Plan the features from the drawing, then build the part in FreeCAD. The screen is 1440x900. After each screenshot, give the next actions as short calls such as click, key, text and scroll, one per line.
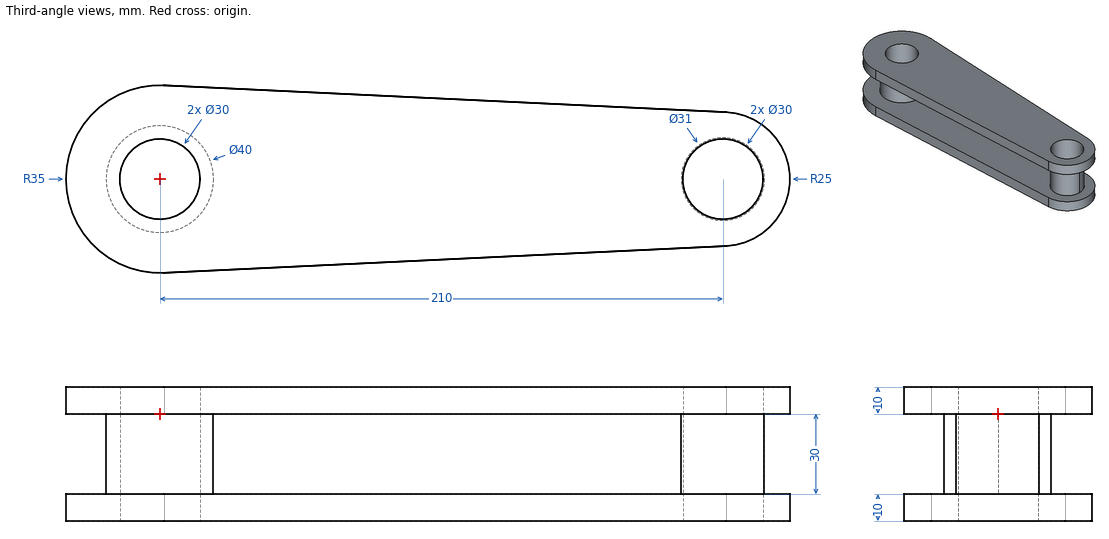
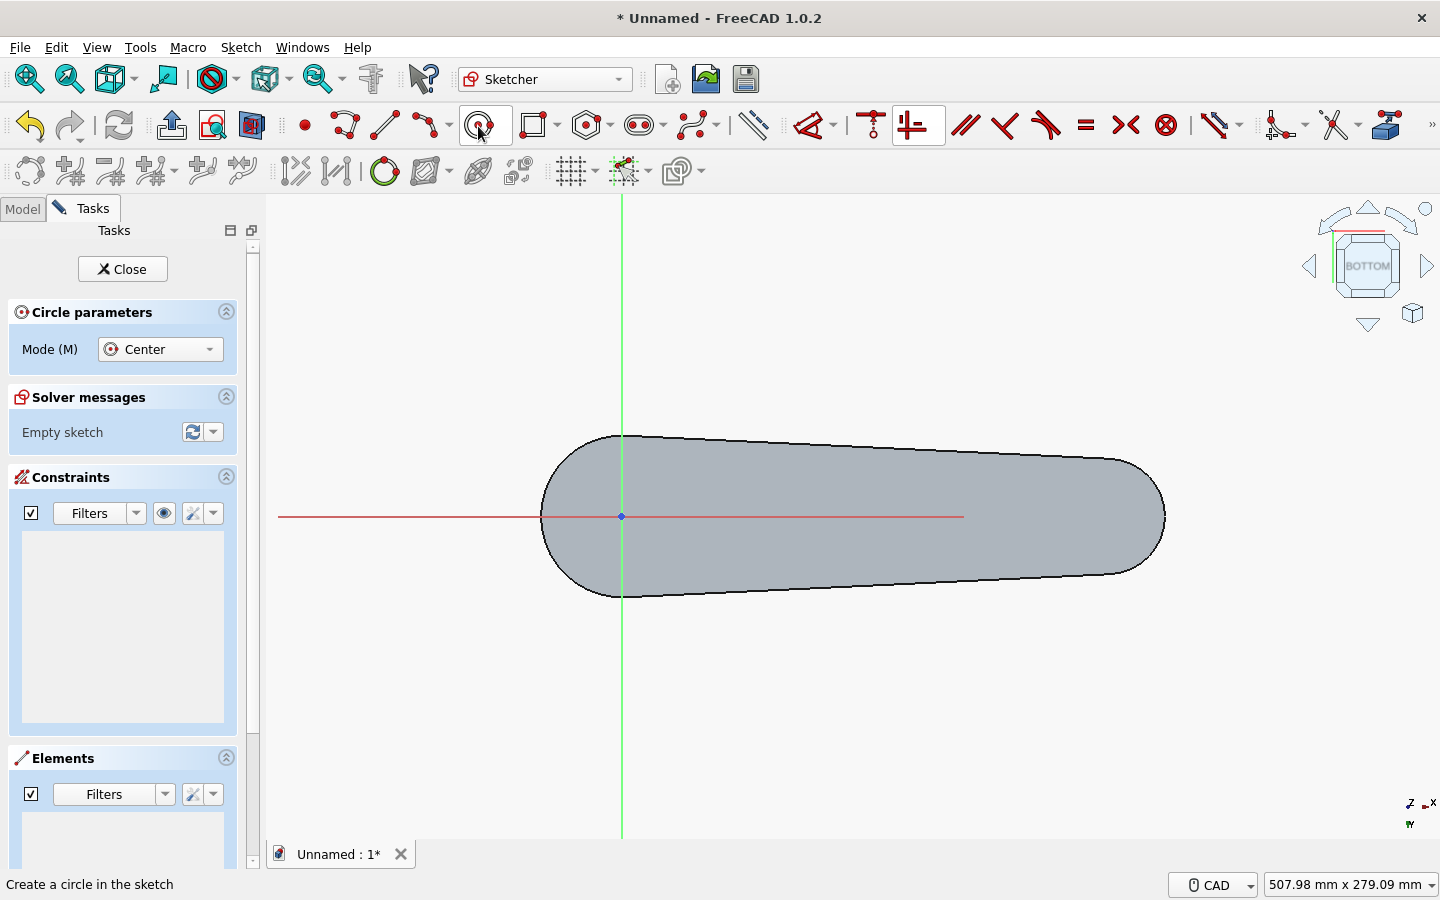
click(622, 516)
move(655, 484)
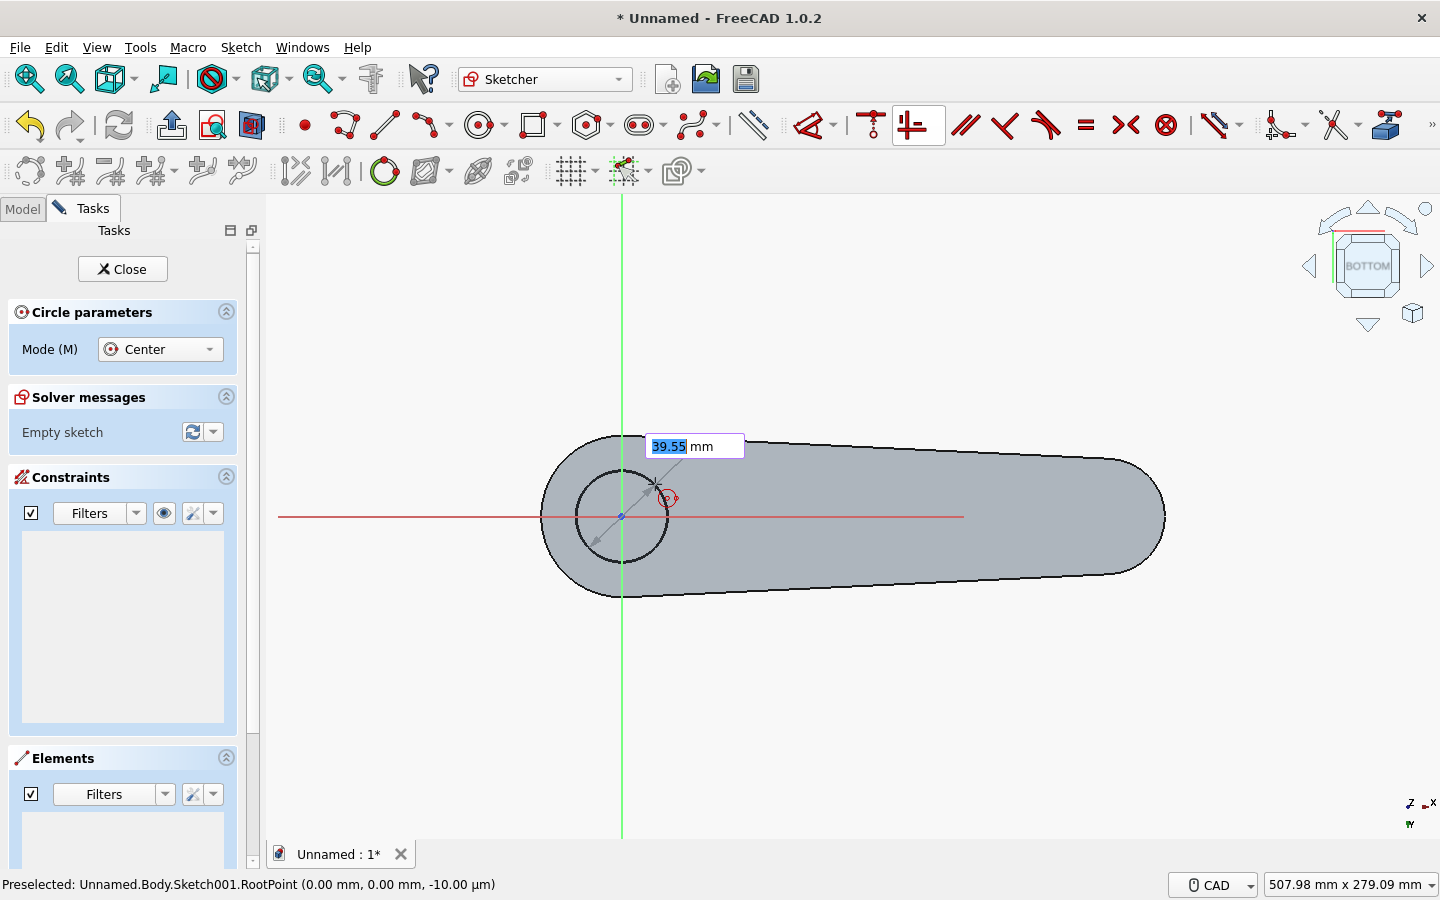
text(40)
key(Return)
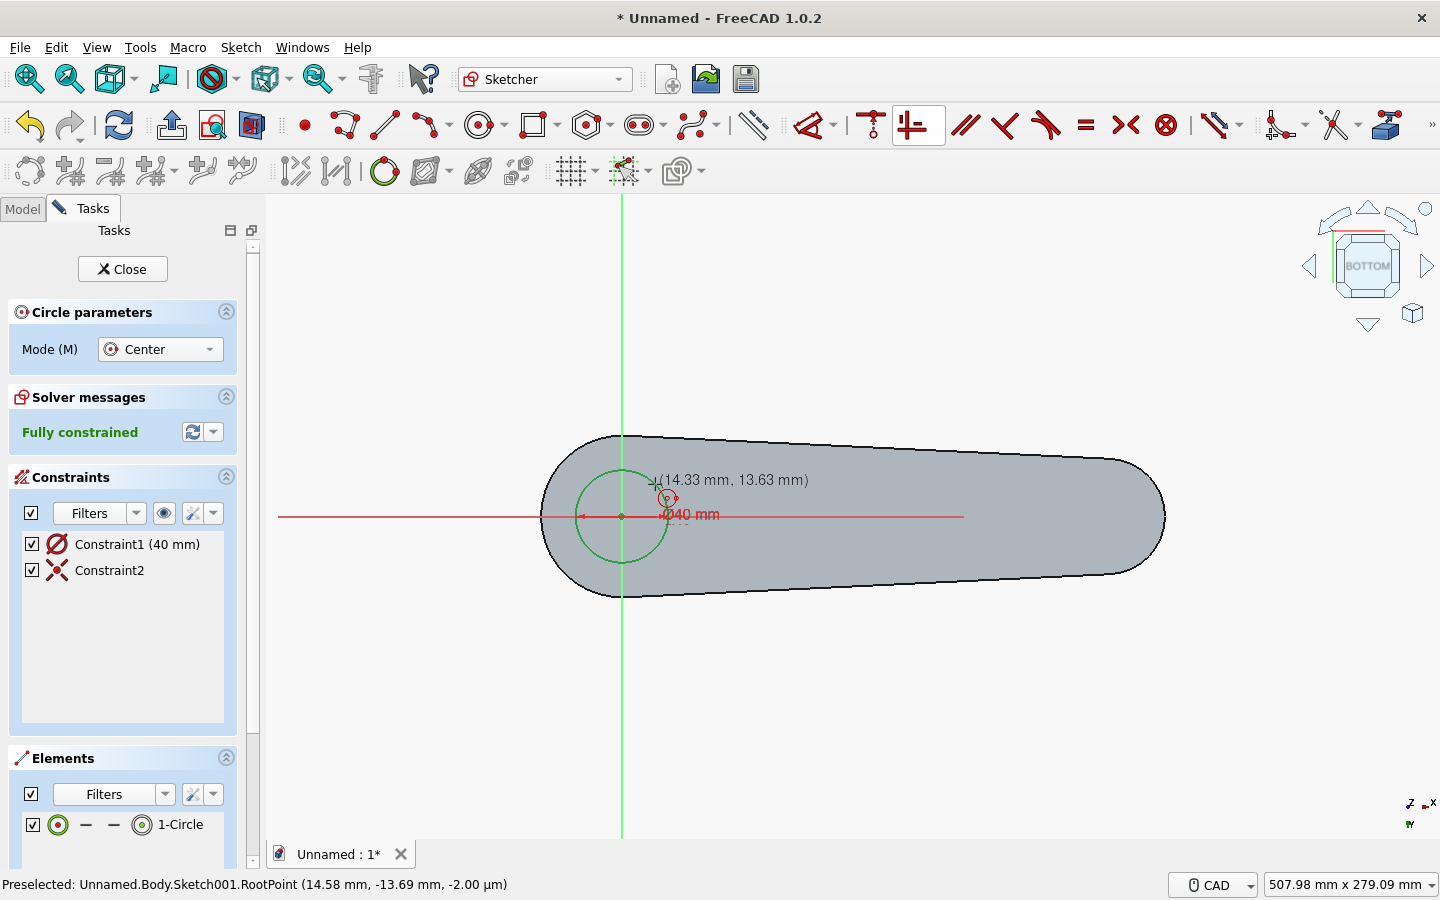
click(1107, 516)
move(1133, 491)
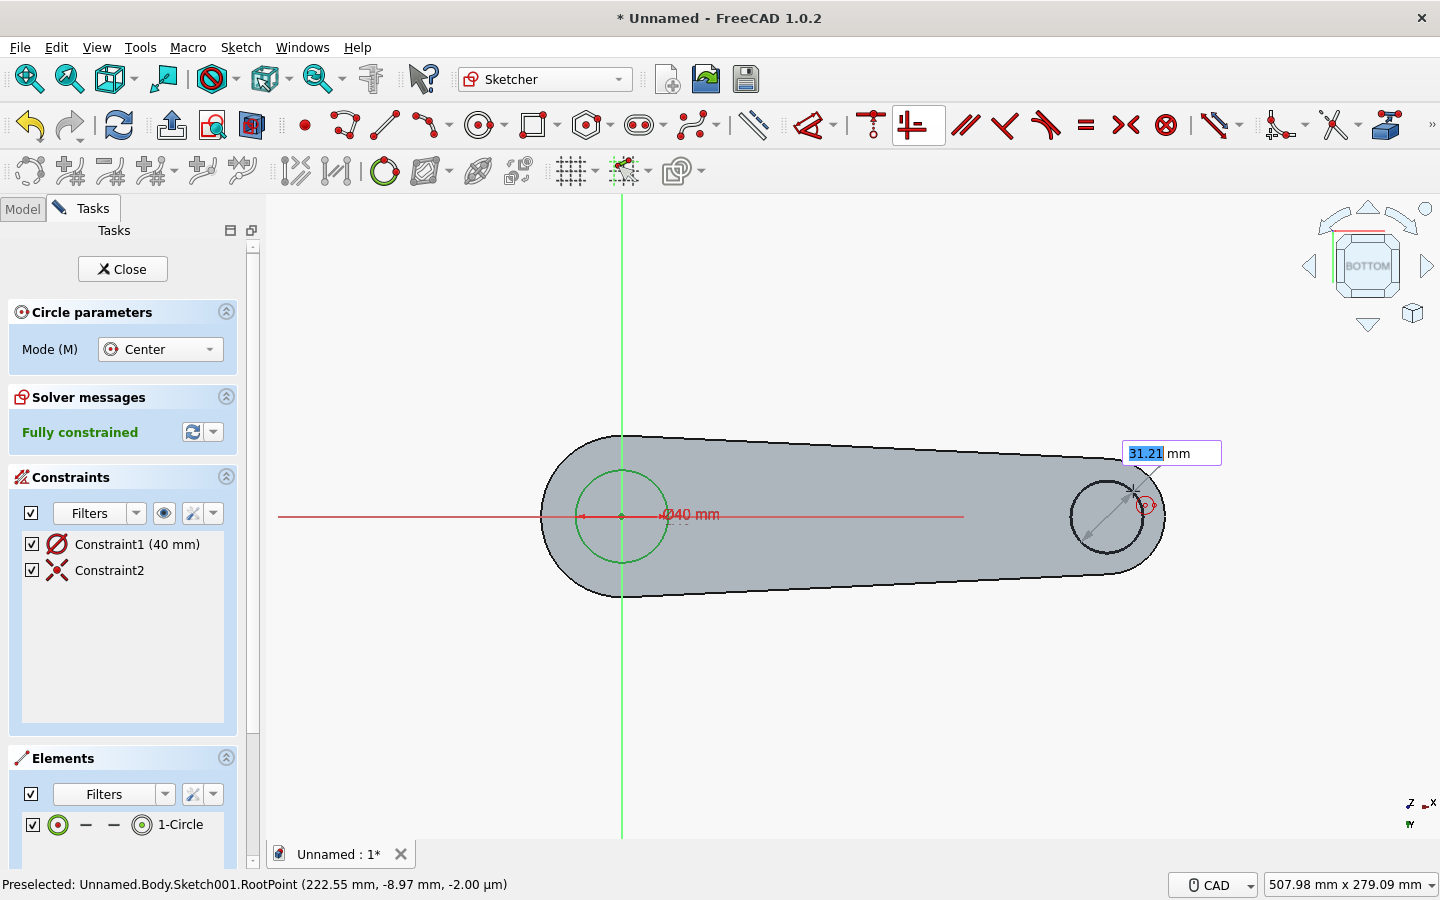
text(31)
key(Return)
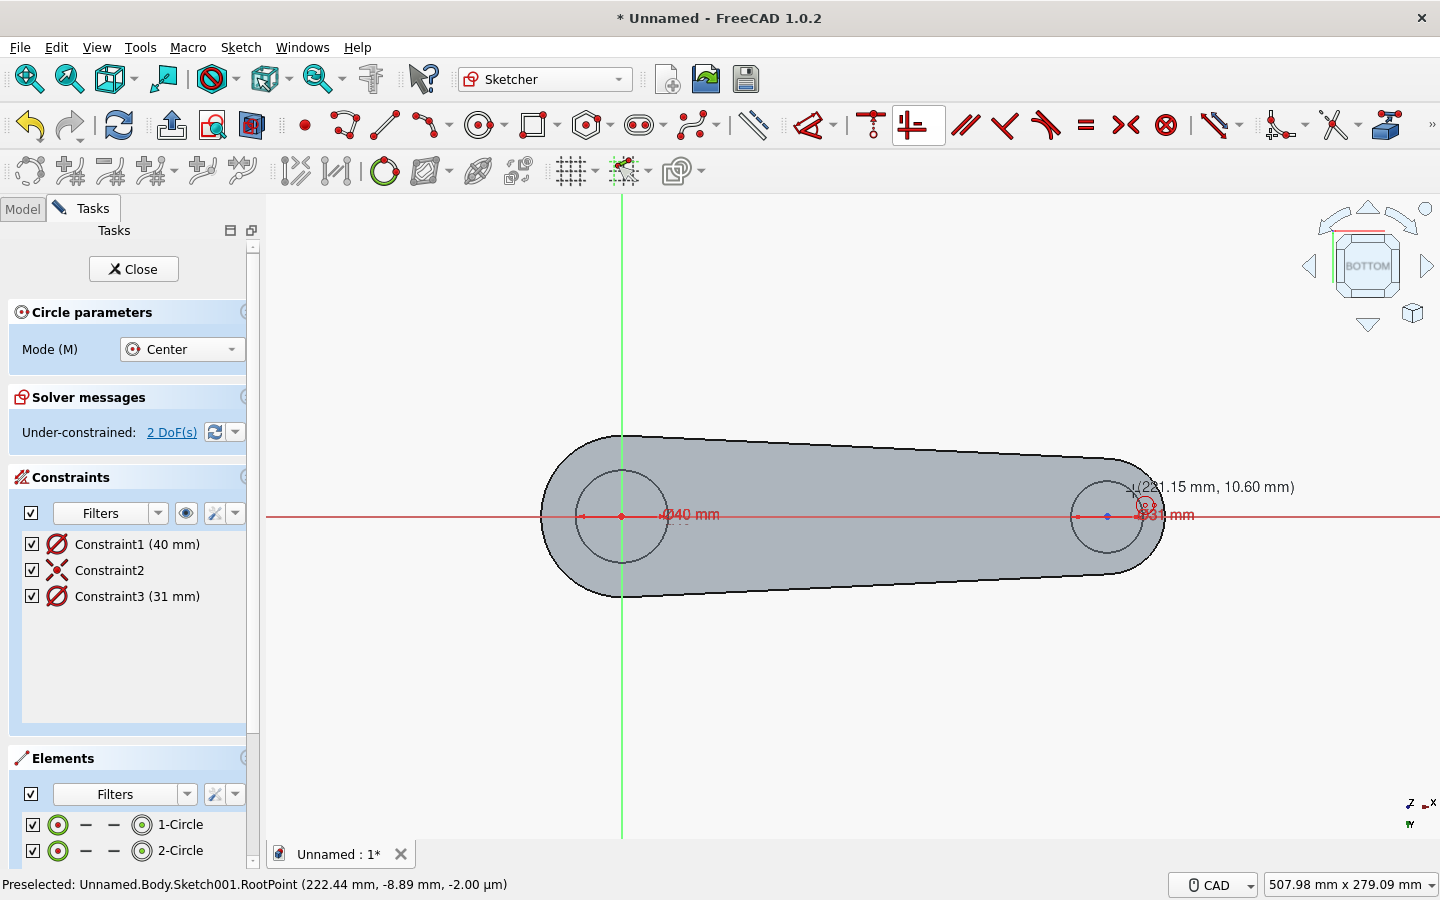
click(622, 516)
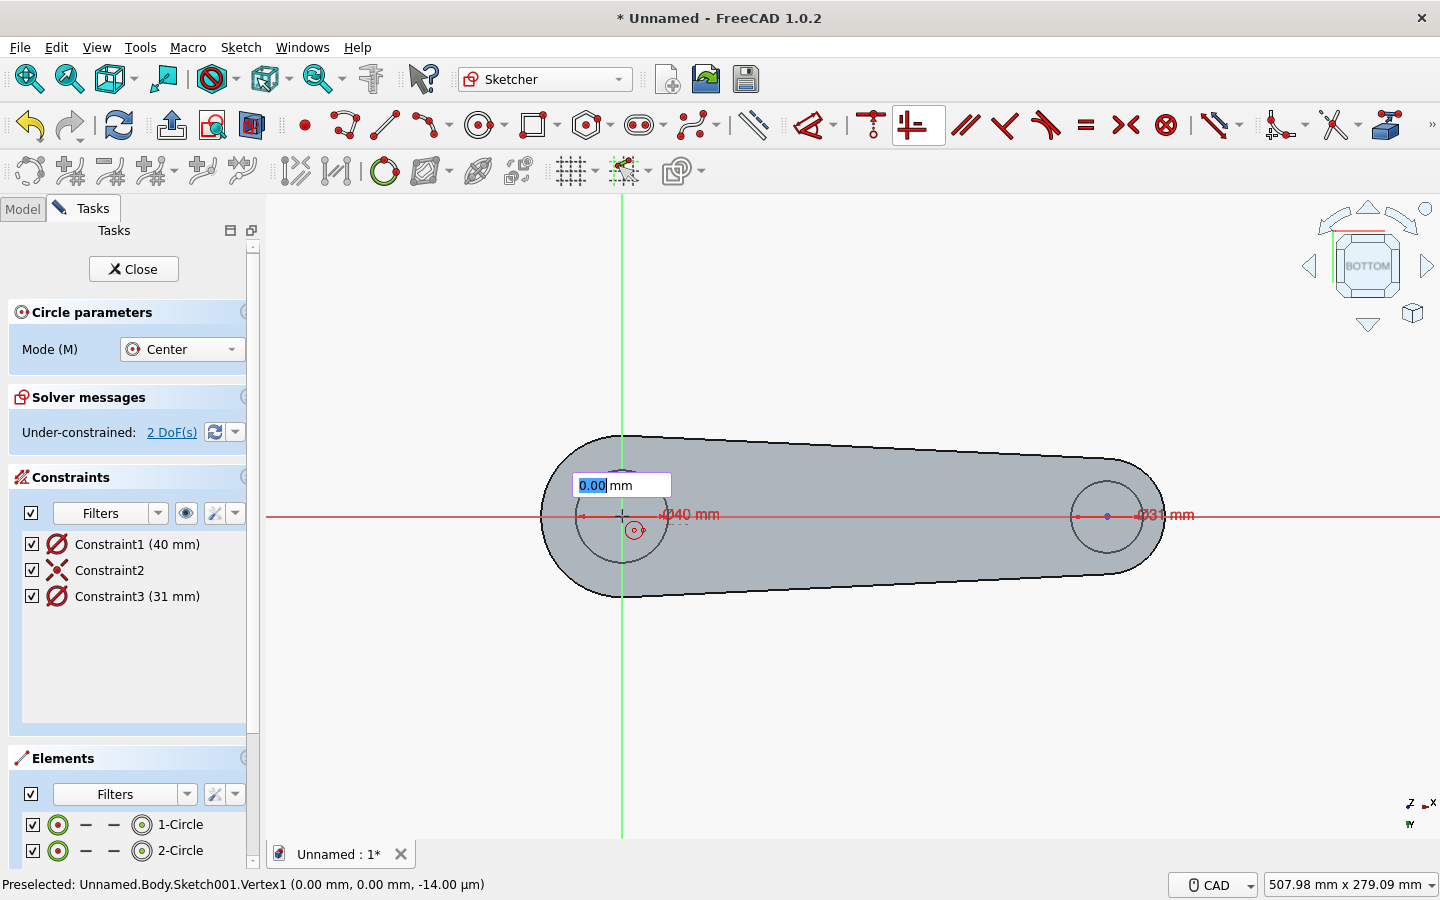
scroll(646, 492, up, 2)
move(646, 492)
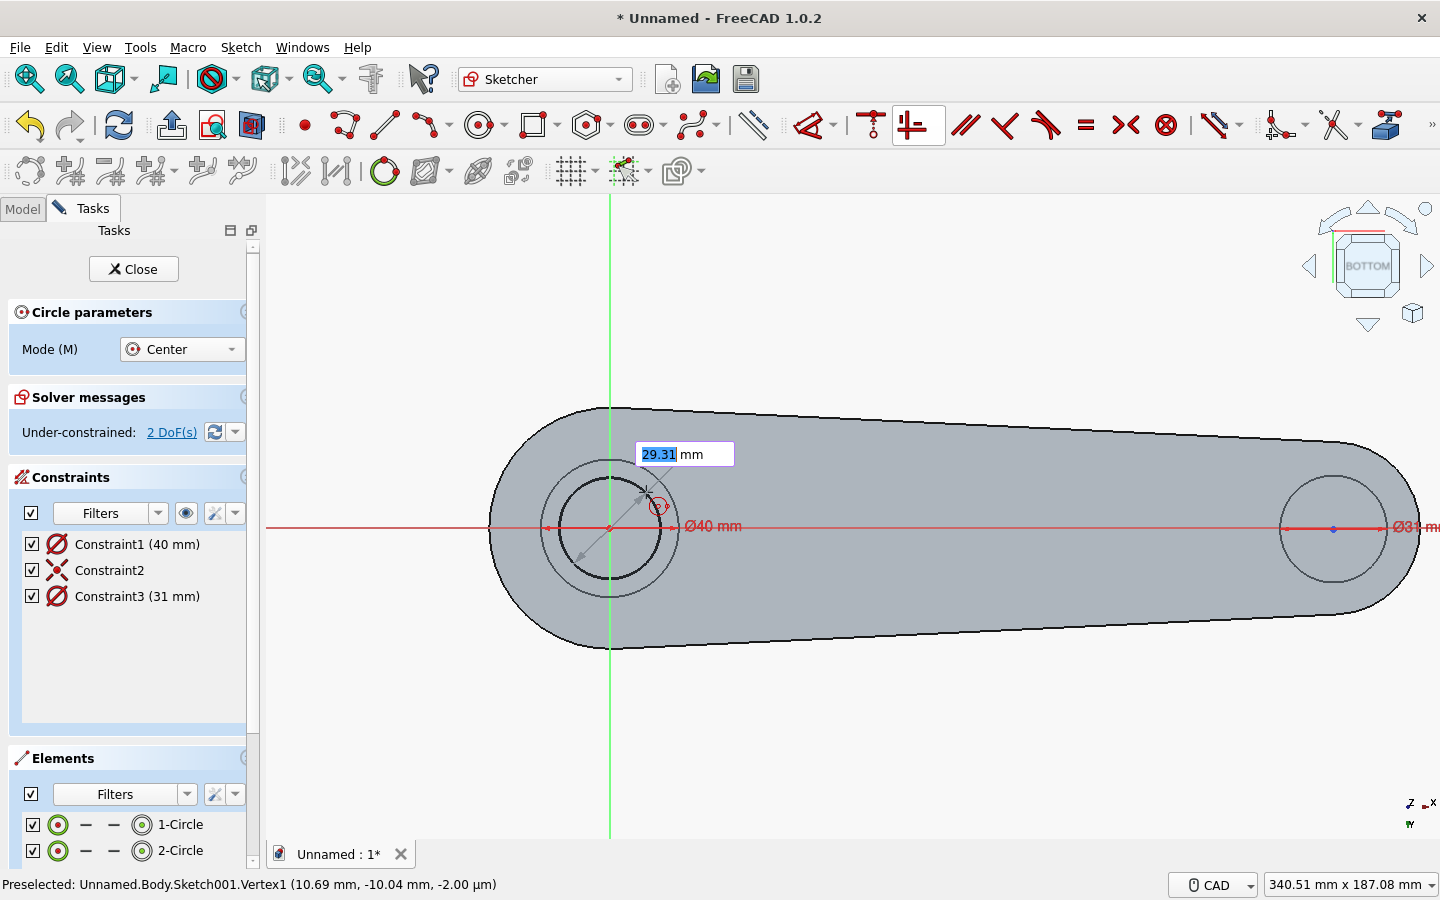
text(30)
key(Return)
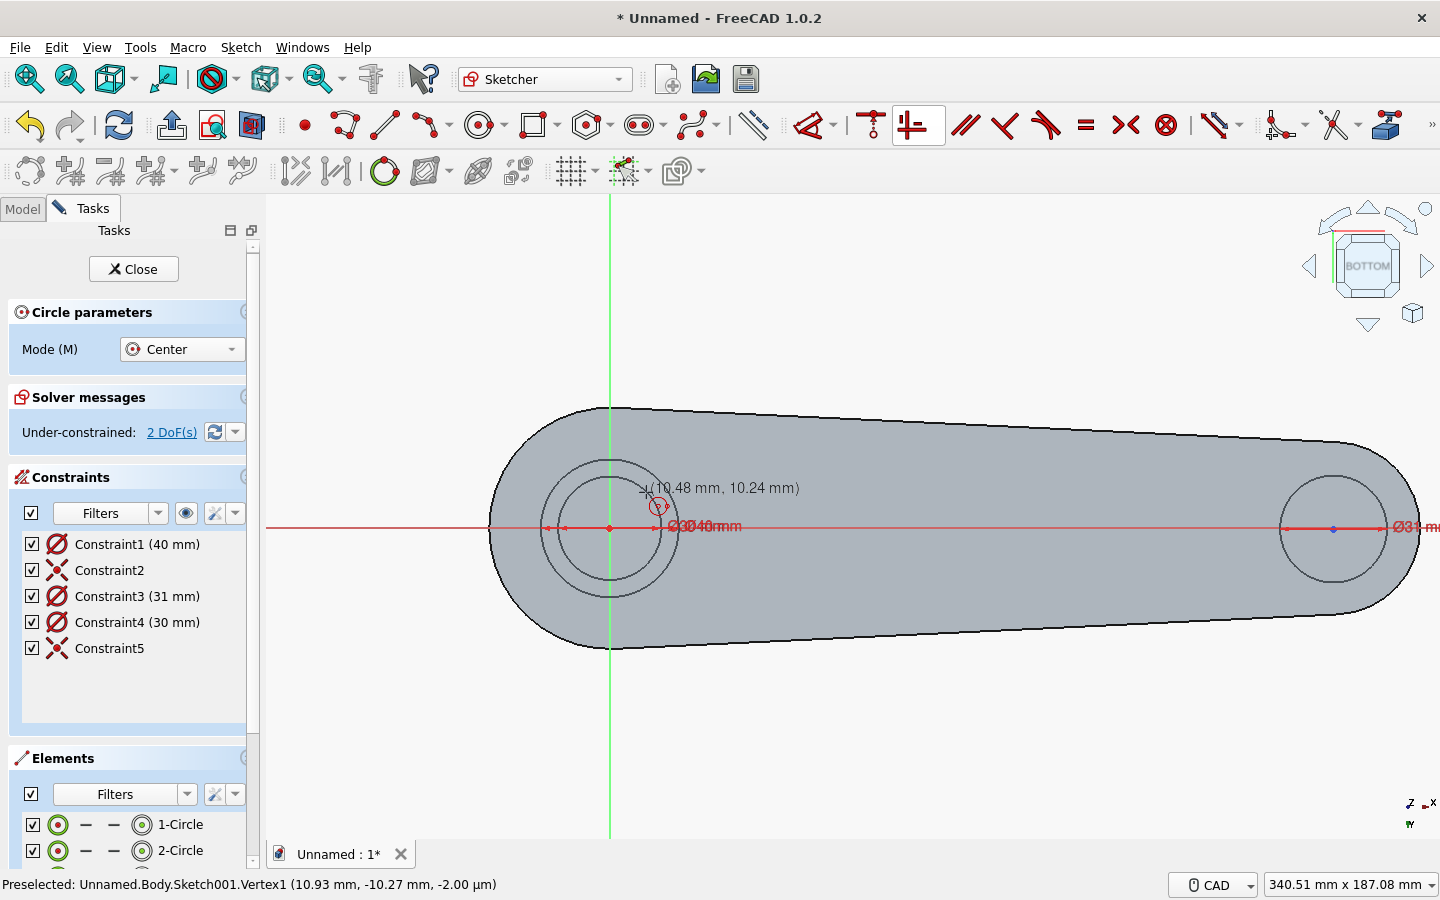
scroll(294, 463, down, 1)